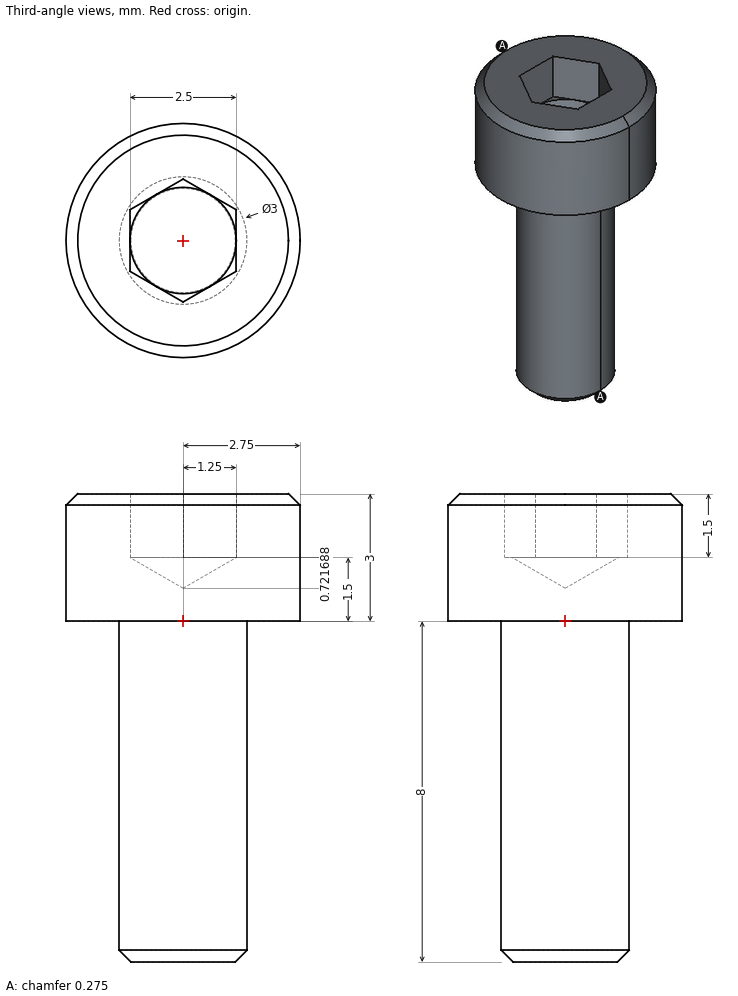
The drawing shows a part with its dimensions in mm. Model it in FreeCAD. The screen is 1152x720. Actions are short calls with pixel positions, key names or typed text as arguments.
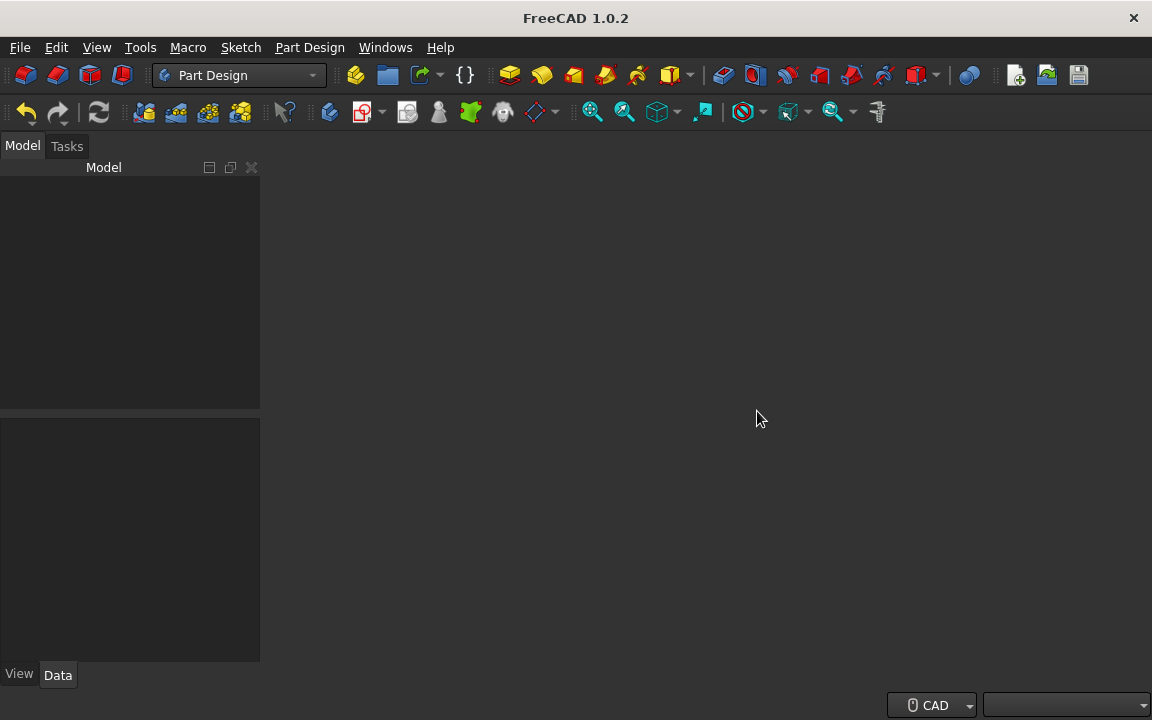
click(1016, 76)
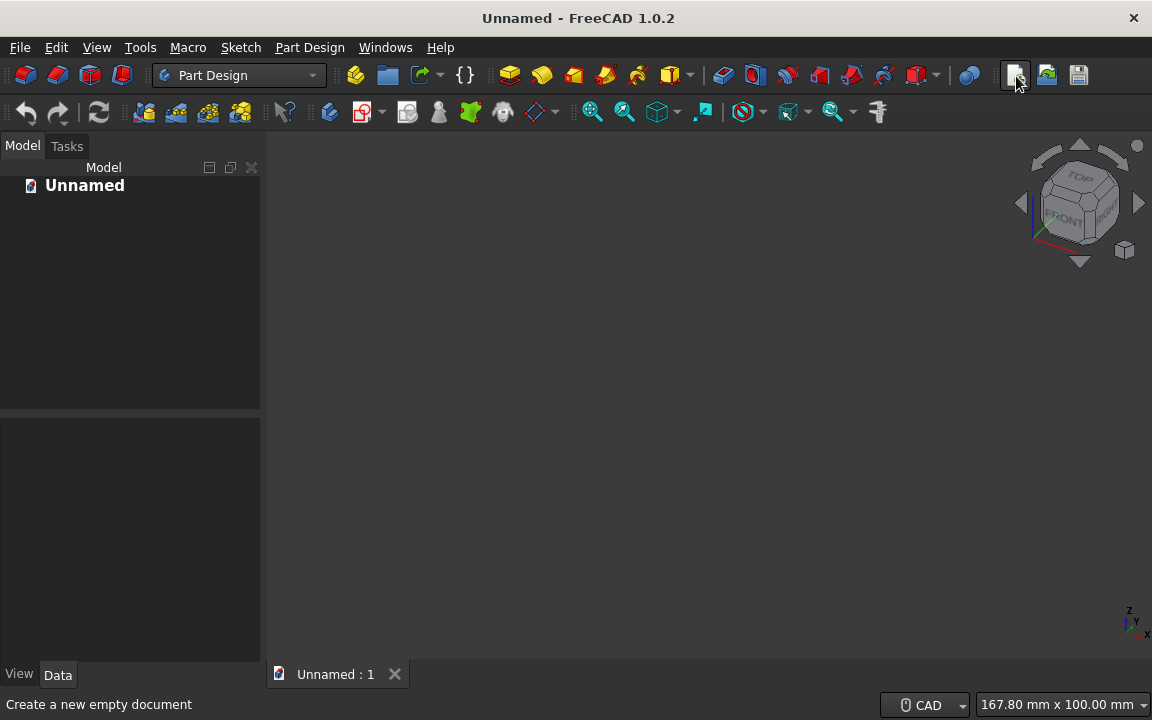
click(362, 112)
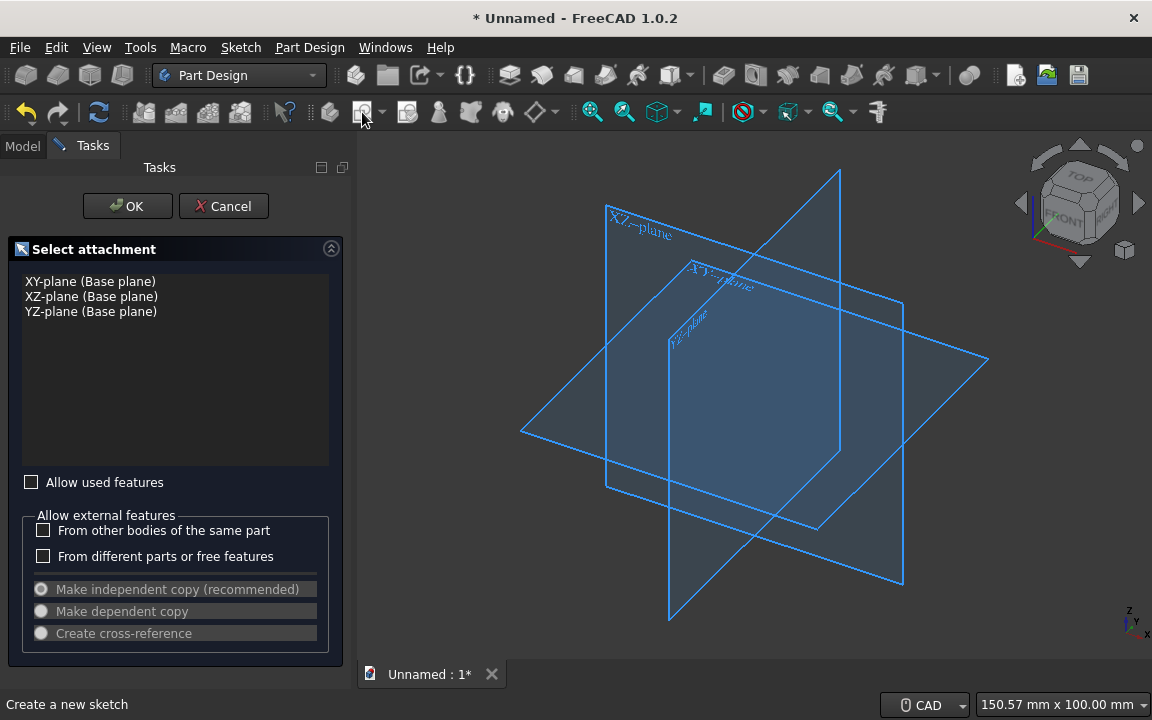
click(82, 296)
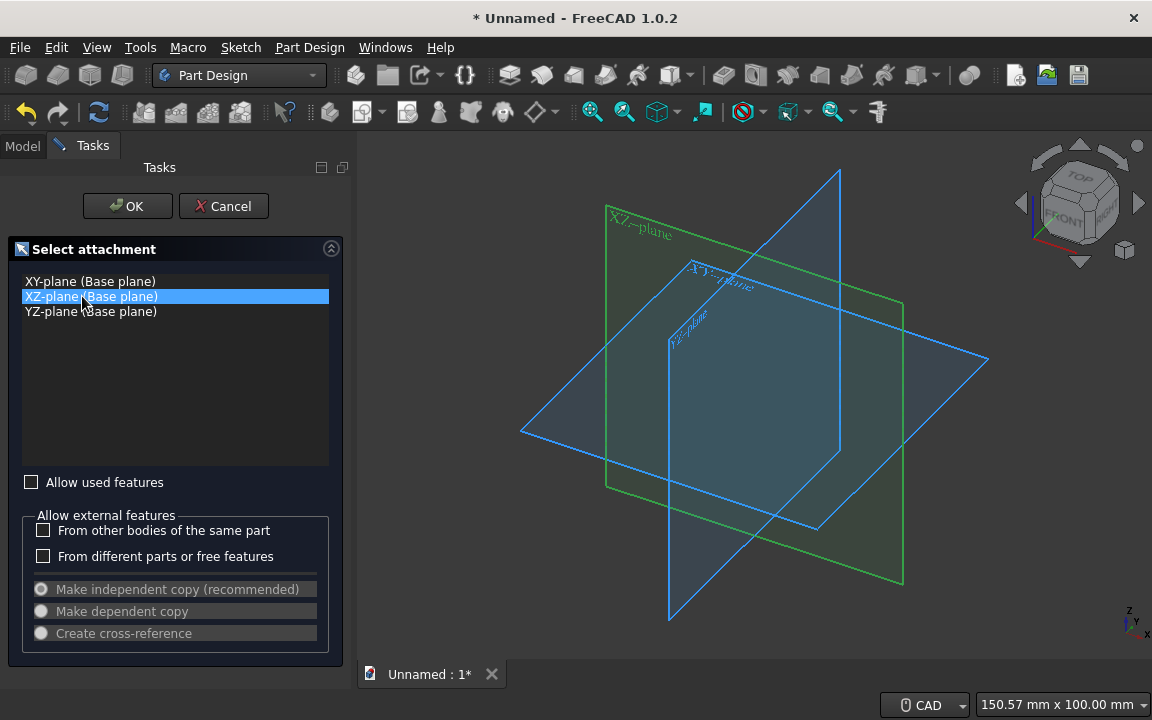
click(128, 206)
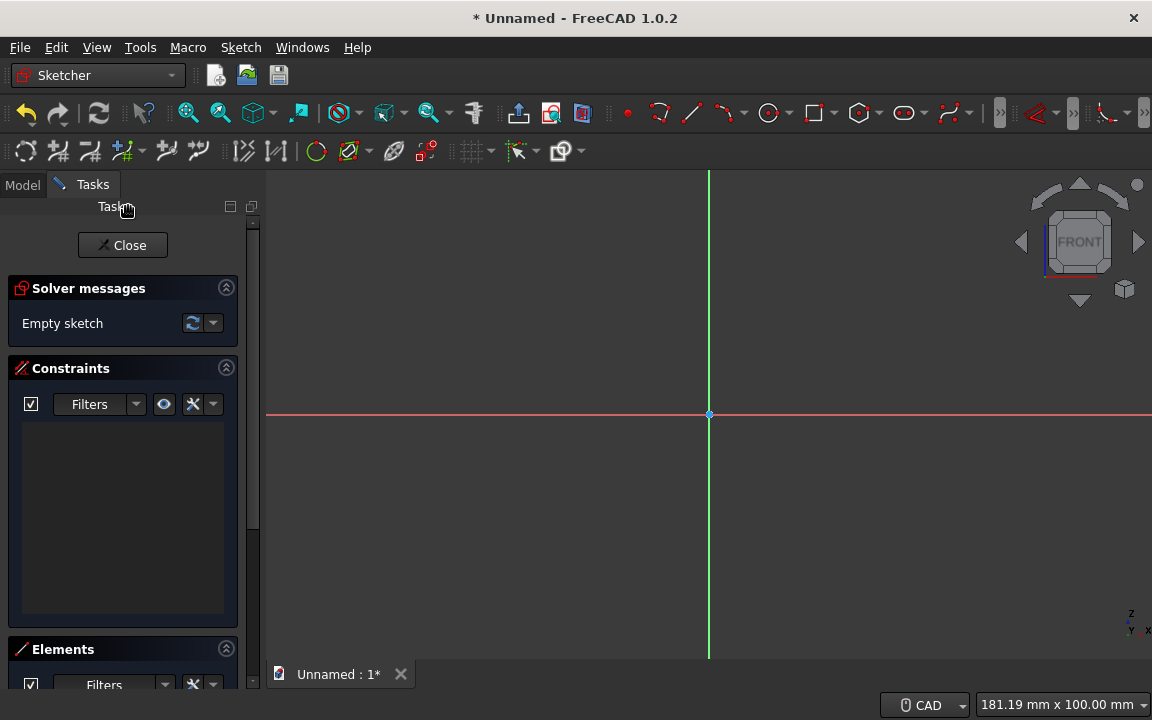
scroll(720, 407, up, 15)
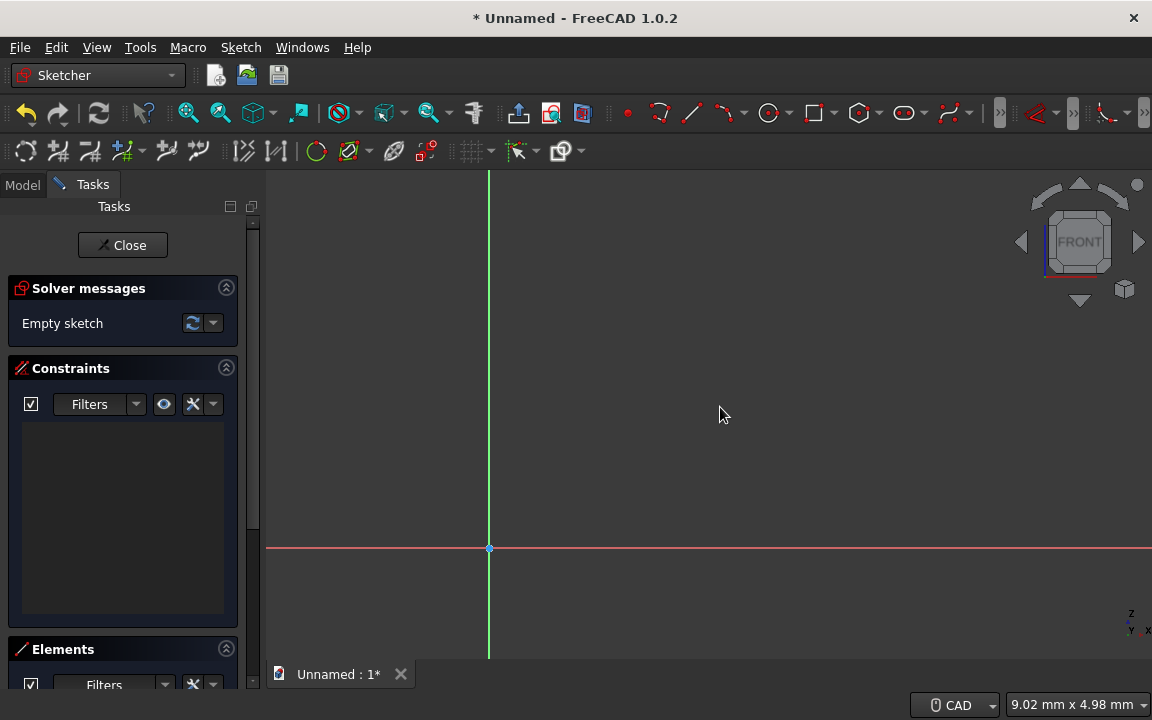
click(814, 114)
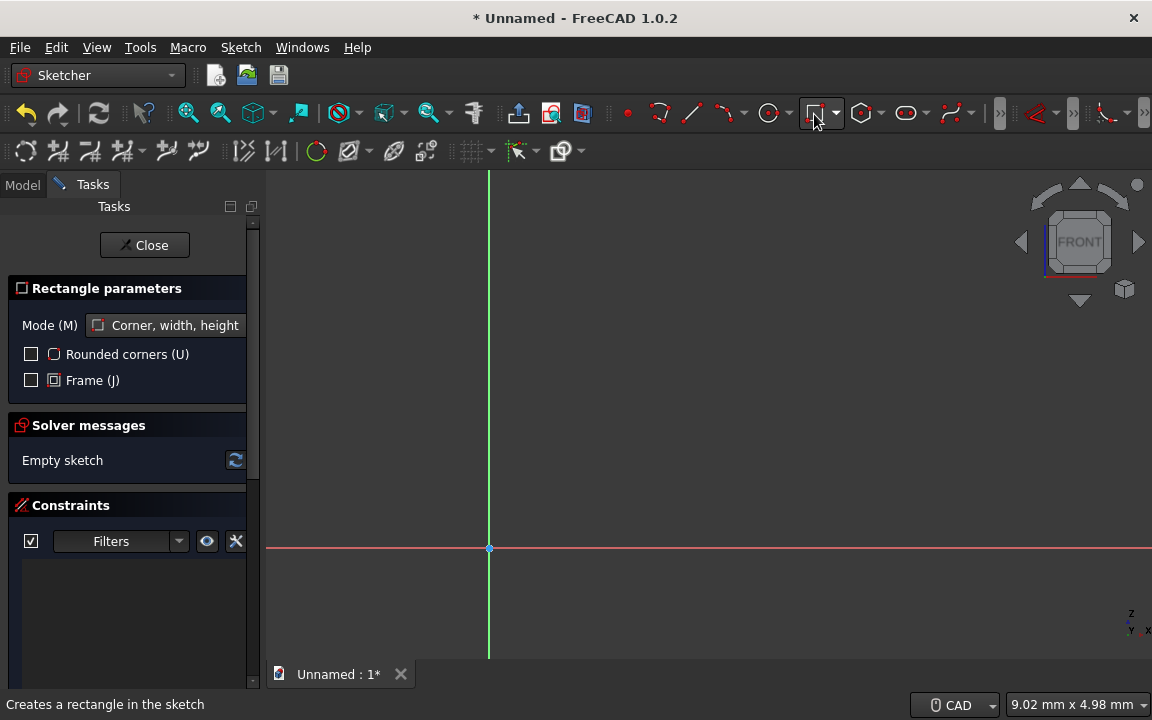
click(489, 548)
move(759, 254)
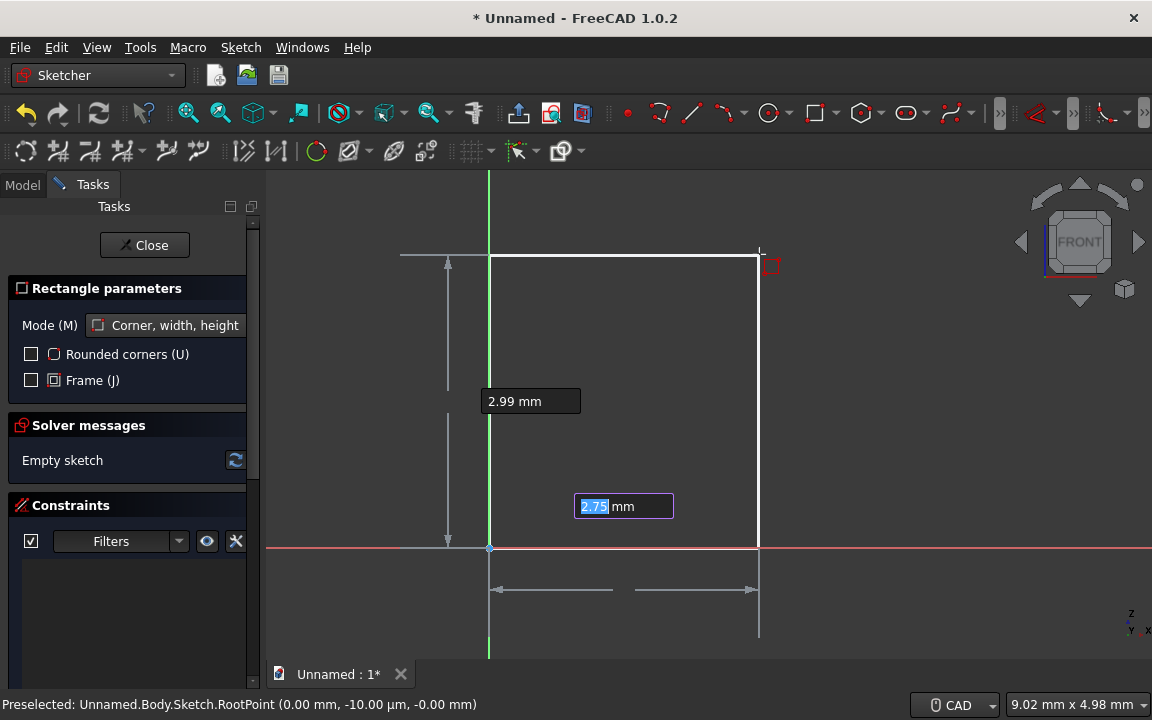
text(2.75)
key(Tab)
text(3)
key(Return)
key(Escape)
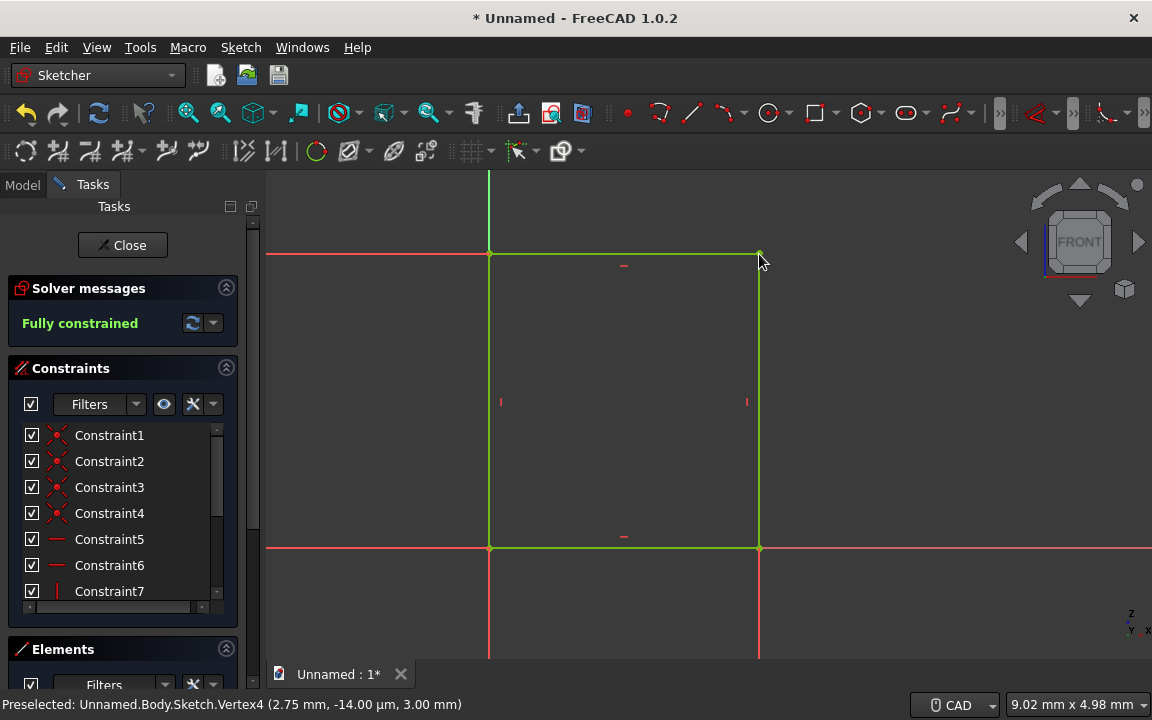
click(123, 245)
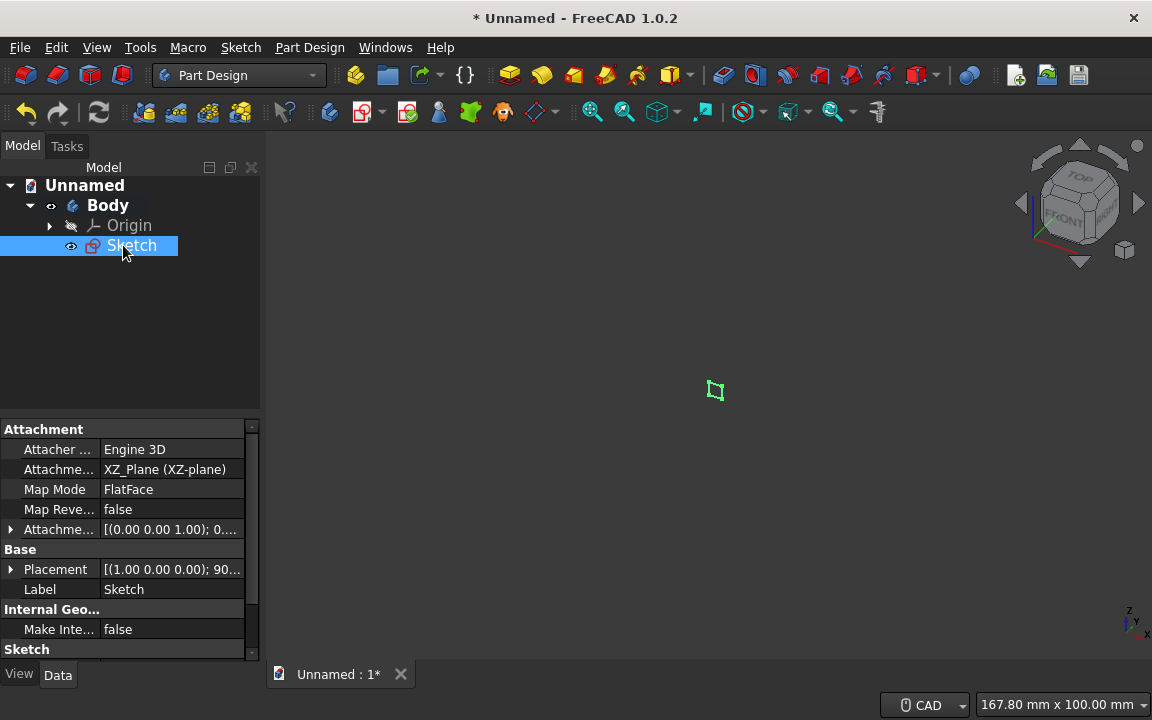
click(542, 76)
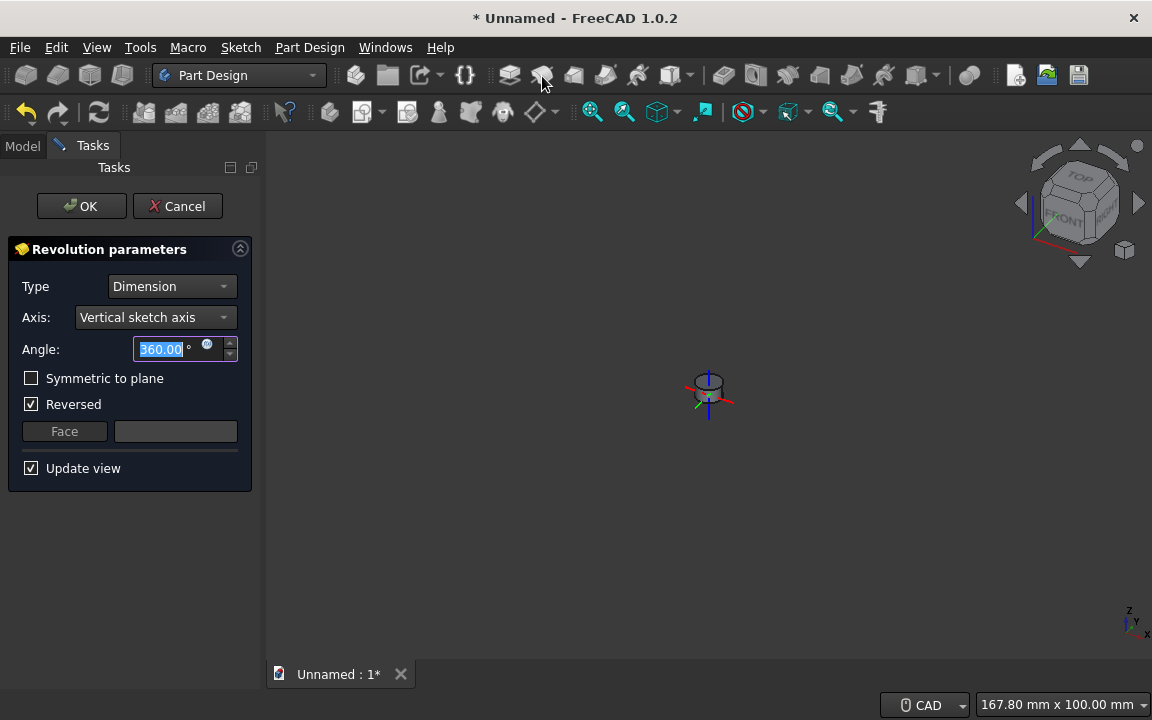
click(82, 206)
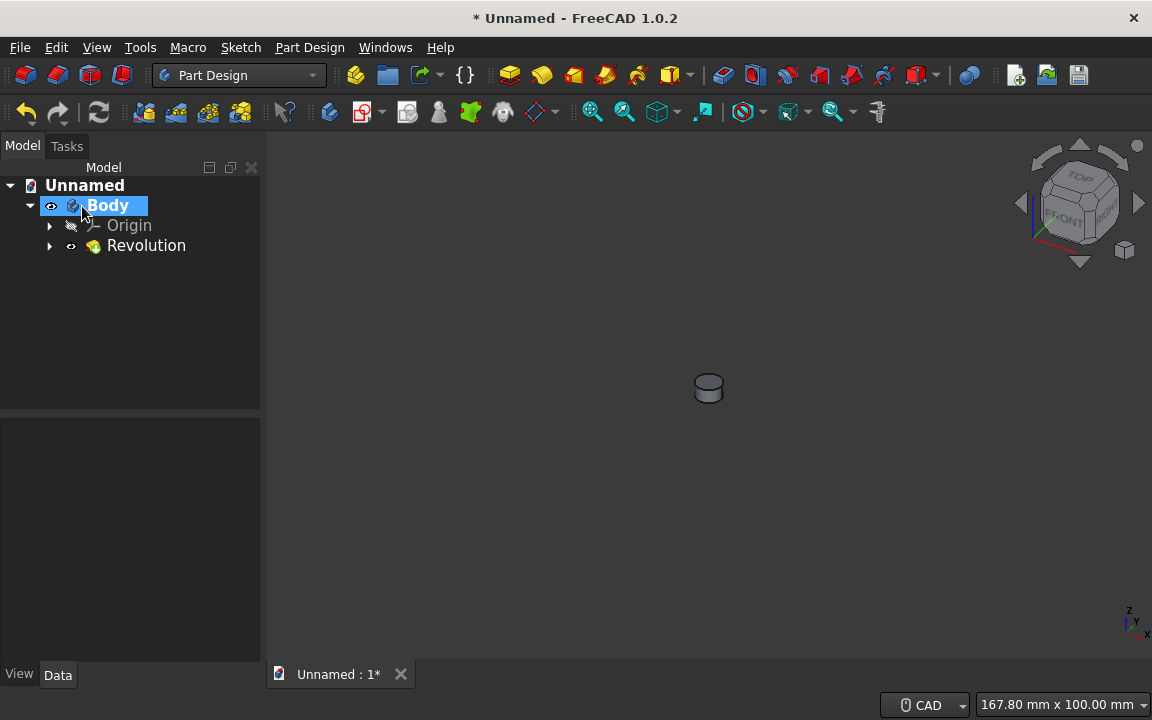
click(594, 112)